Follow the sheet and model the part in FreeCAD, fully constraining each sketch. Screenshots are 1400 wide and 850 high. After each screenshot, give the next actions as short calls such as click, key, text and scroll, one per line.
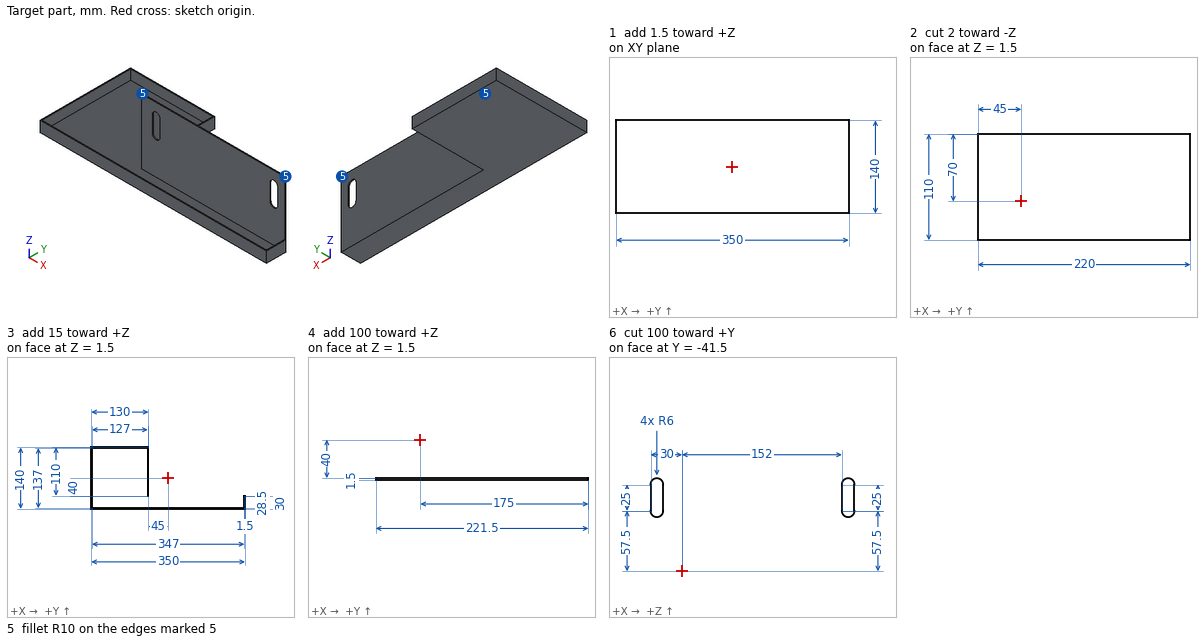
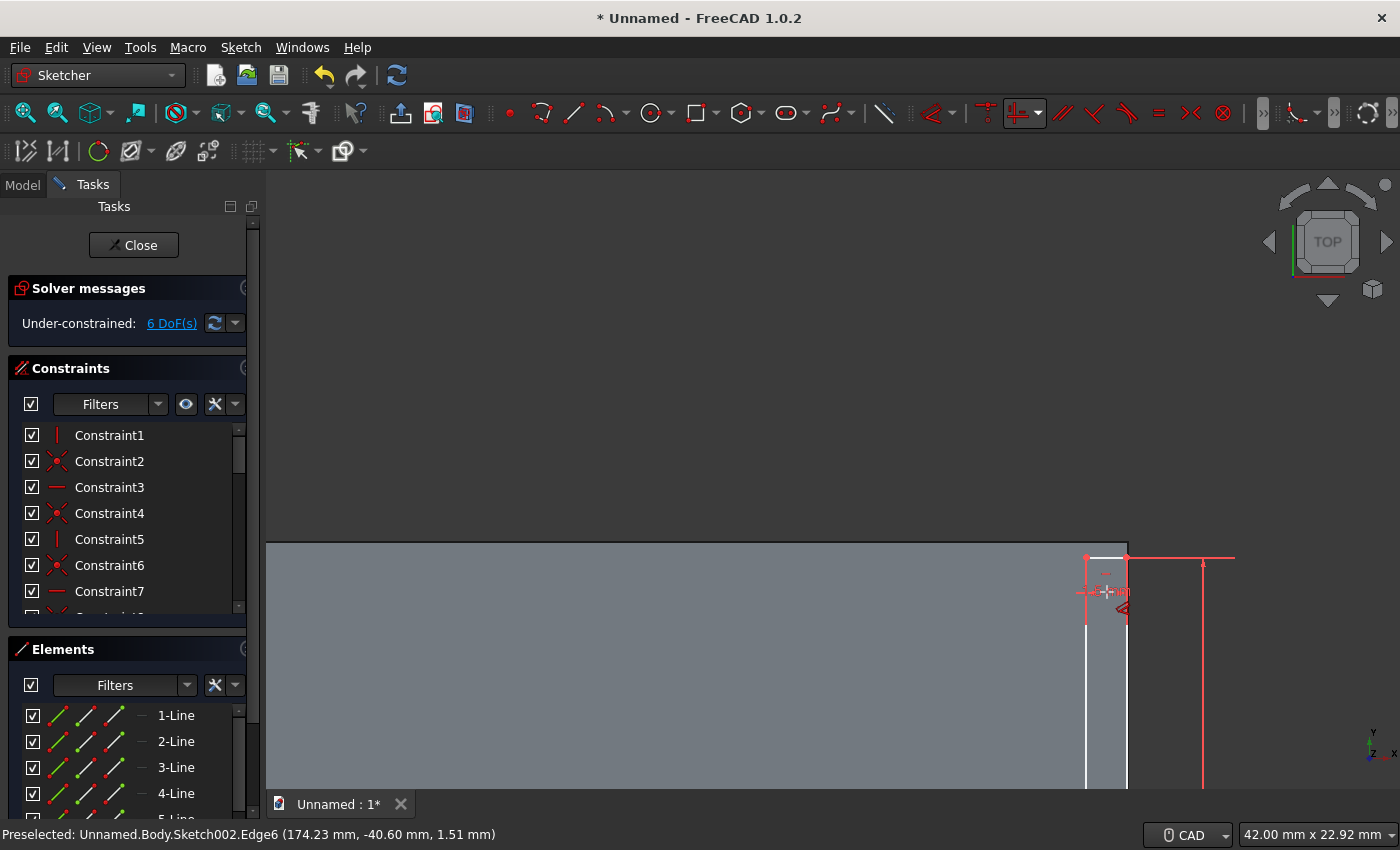
scroll(1114, 561, down, 13)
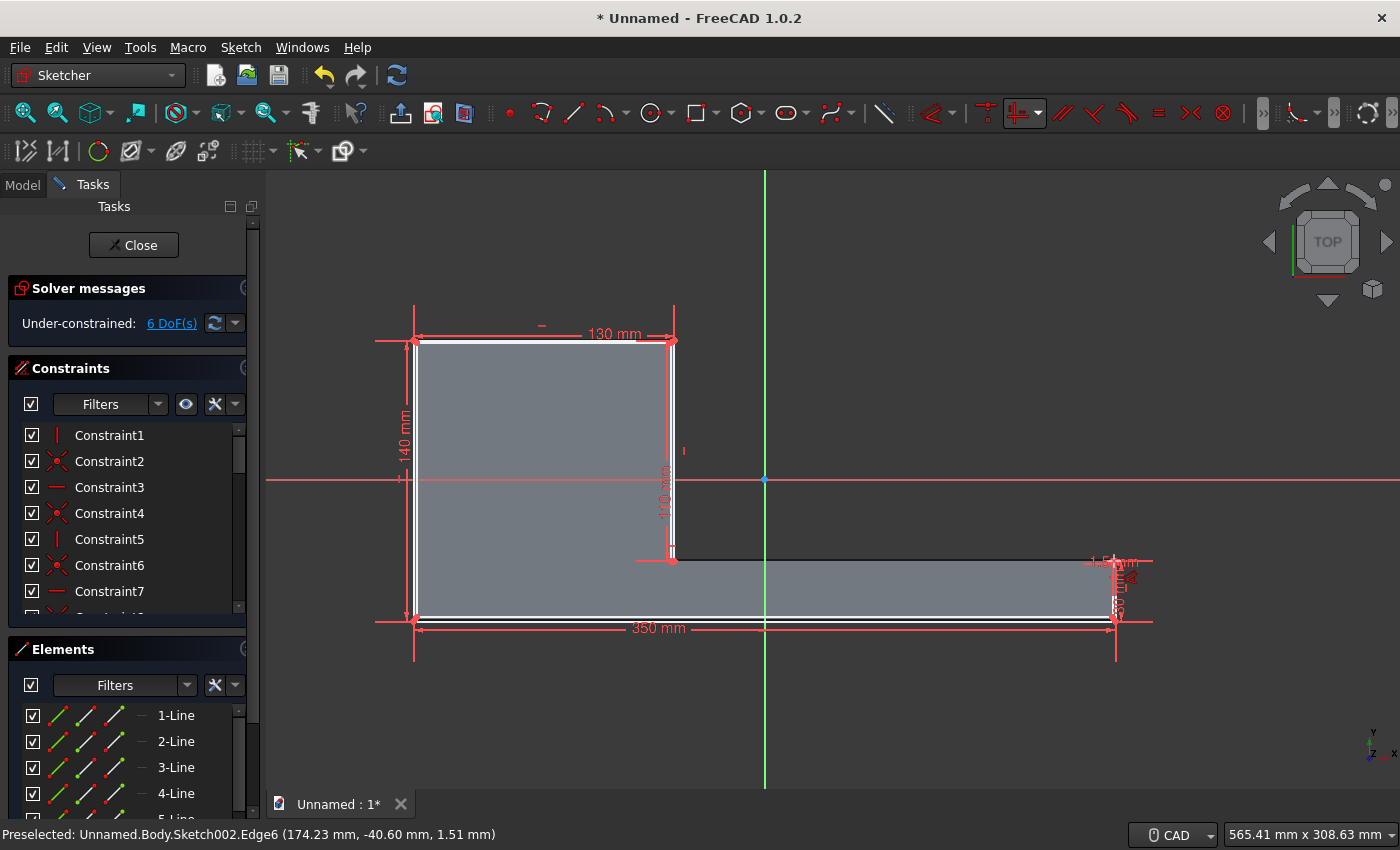
scroll(904, 617, up, 7)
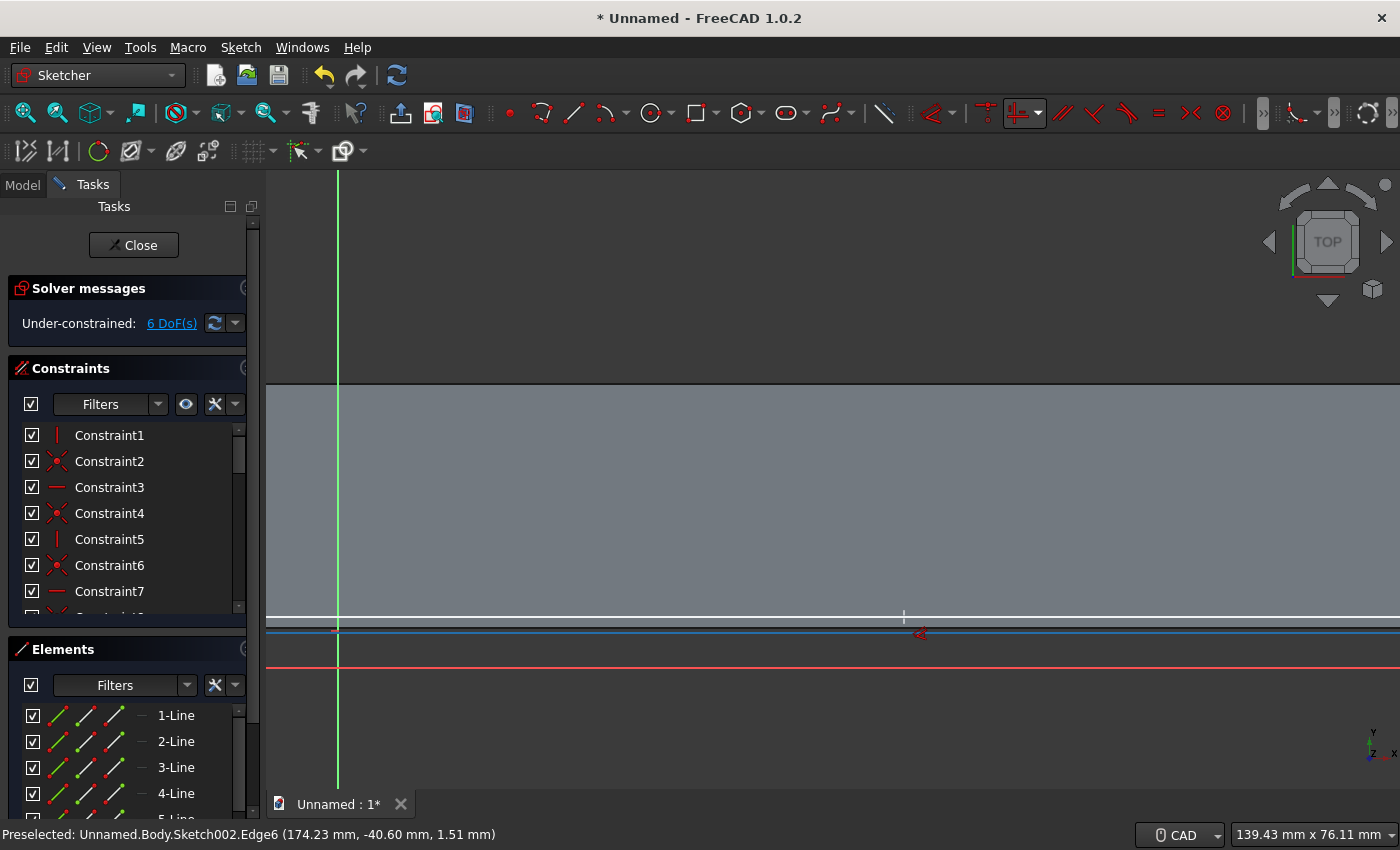
click(902, 617)
click(764, 651)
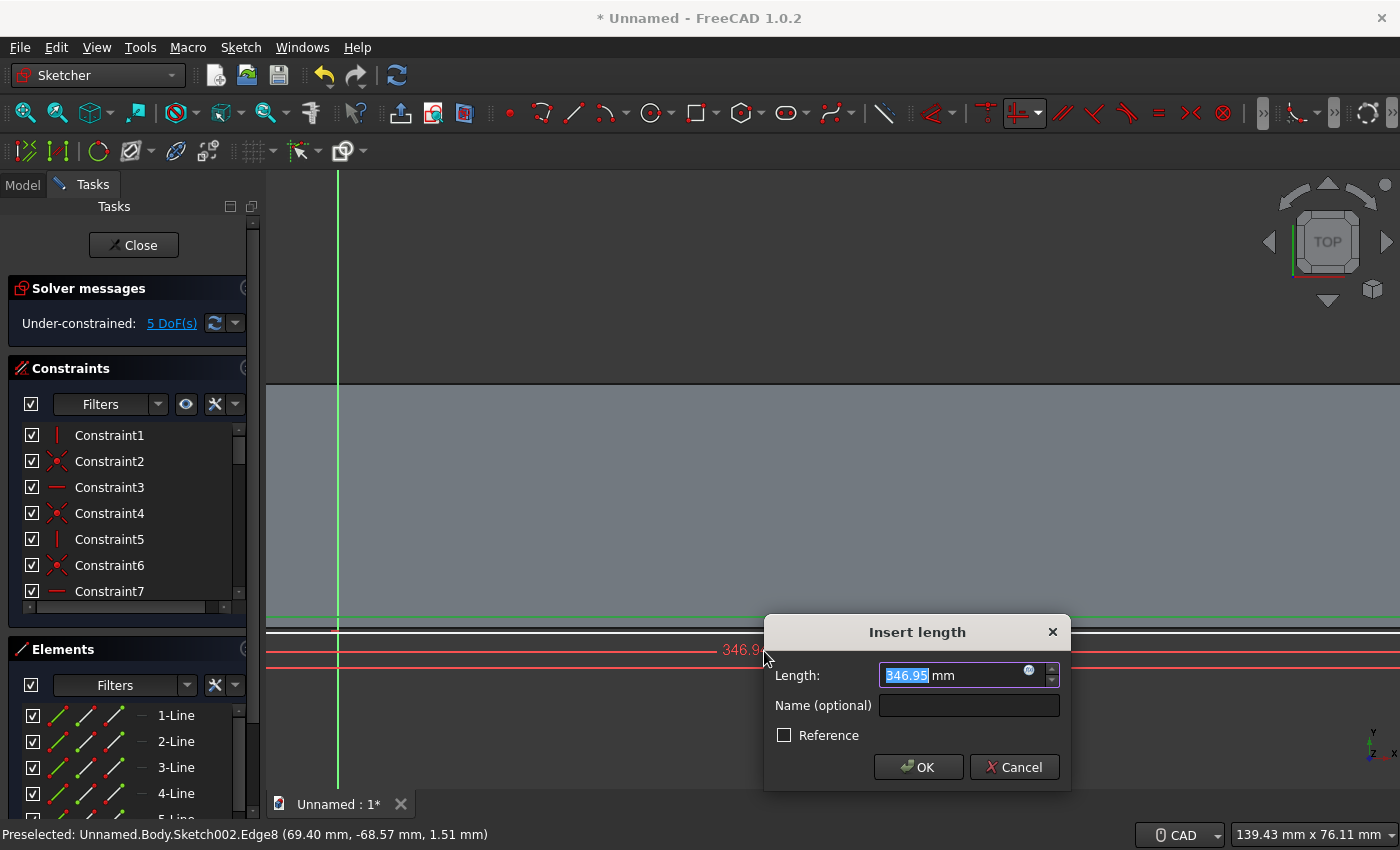
text(347)
key(Return)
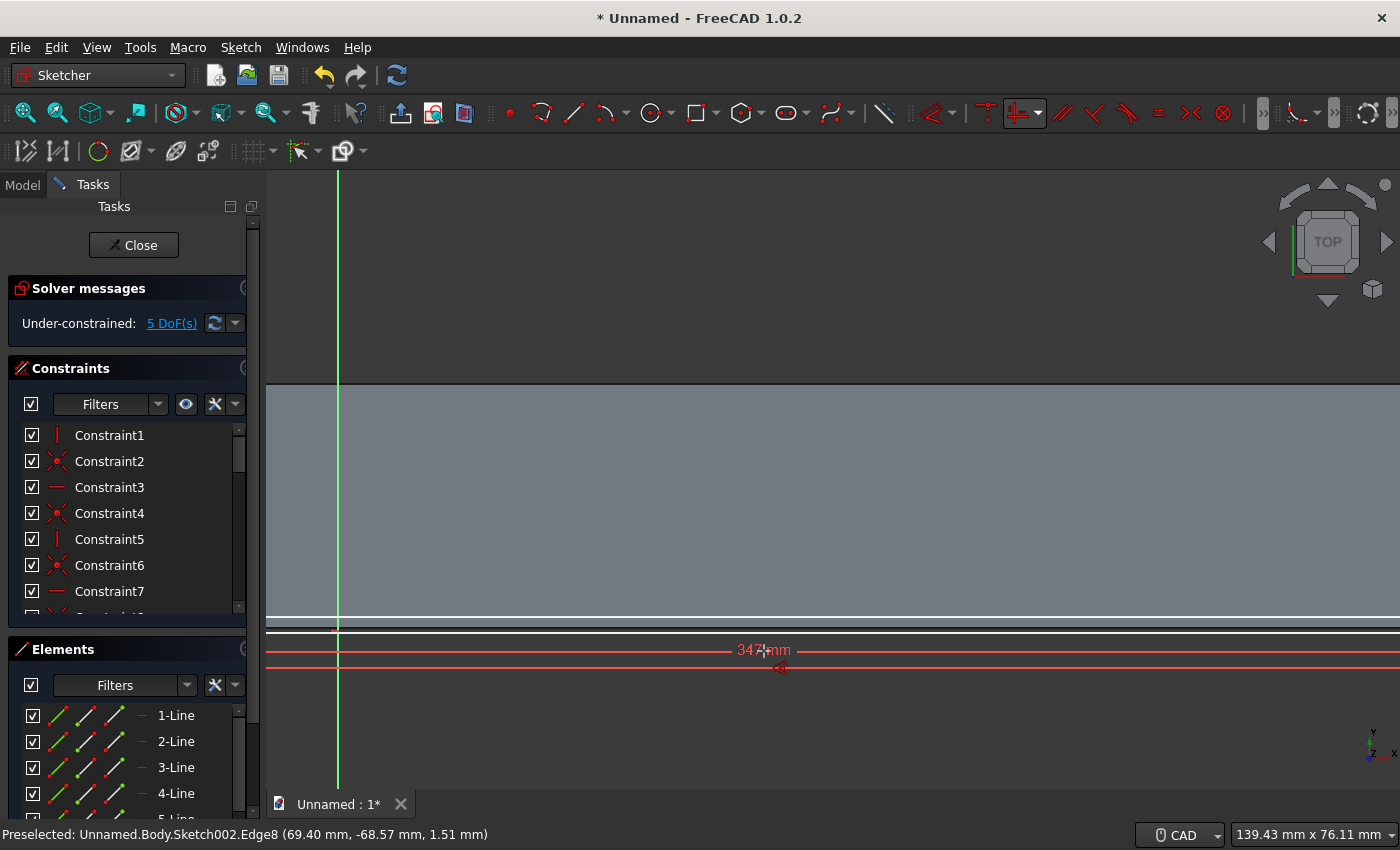
scroll(904, 617, down, 7)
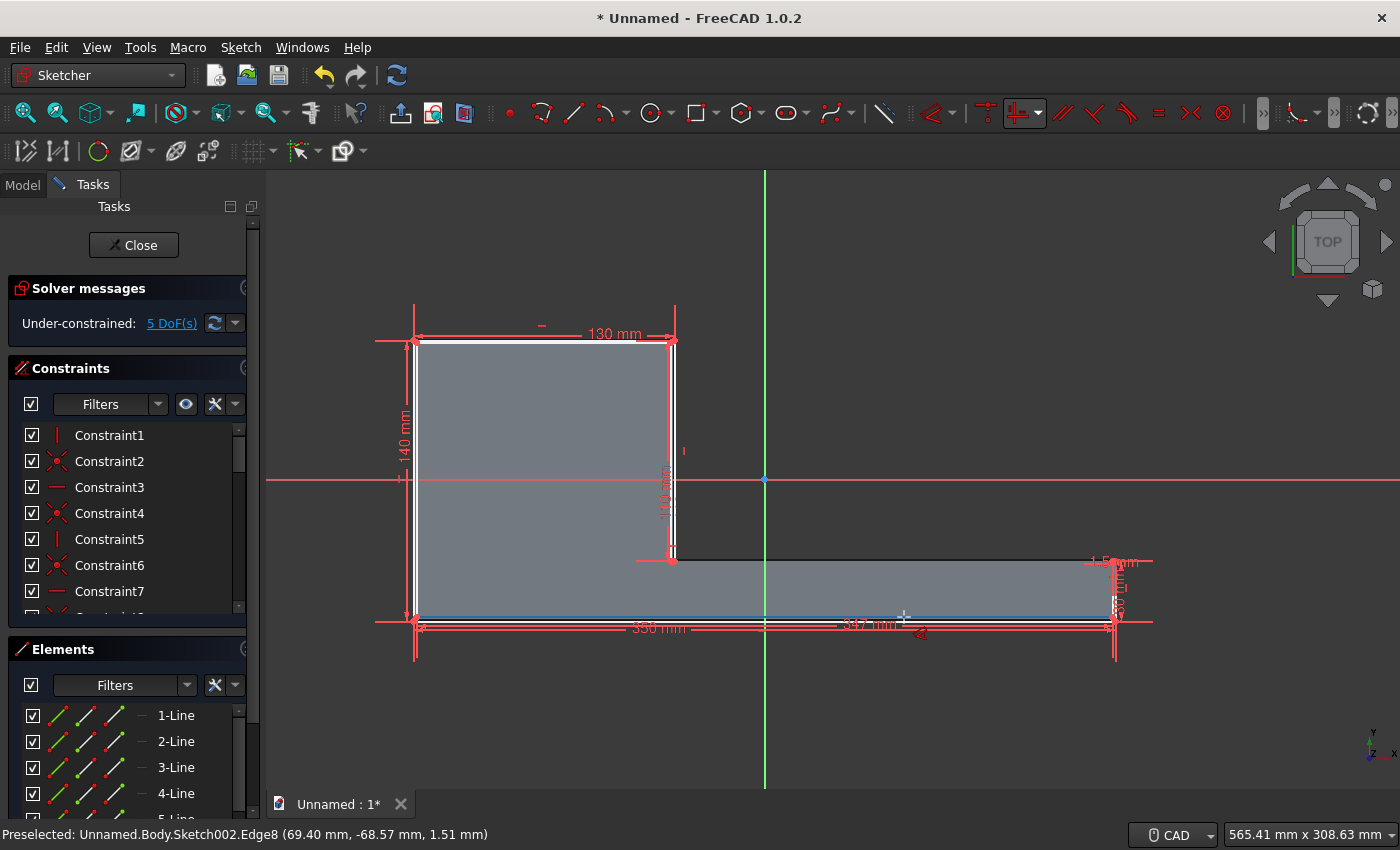
scroll(417, 535, up, 8)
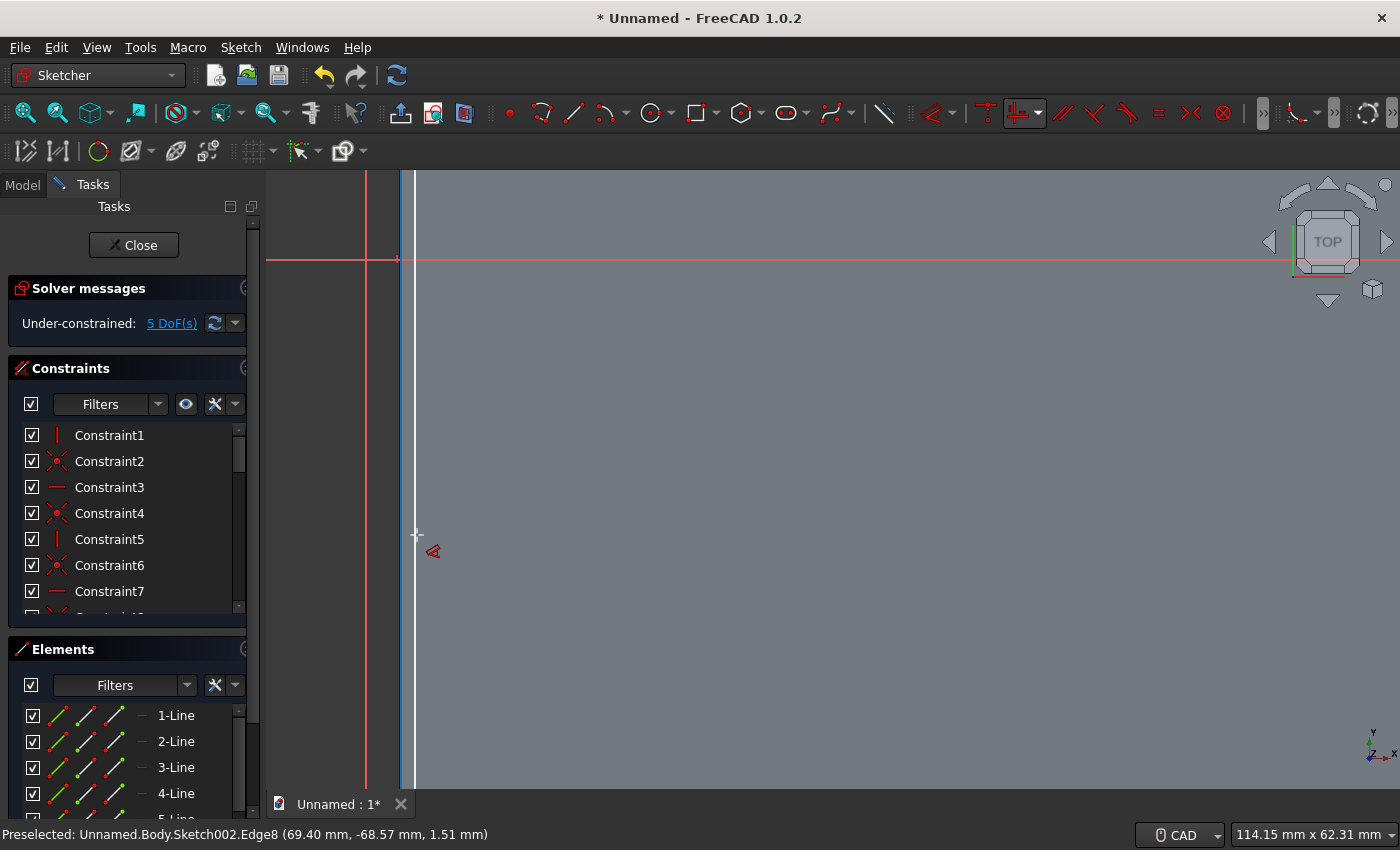
click(415, 533)
click(381, 480)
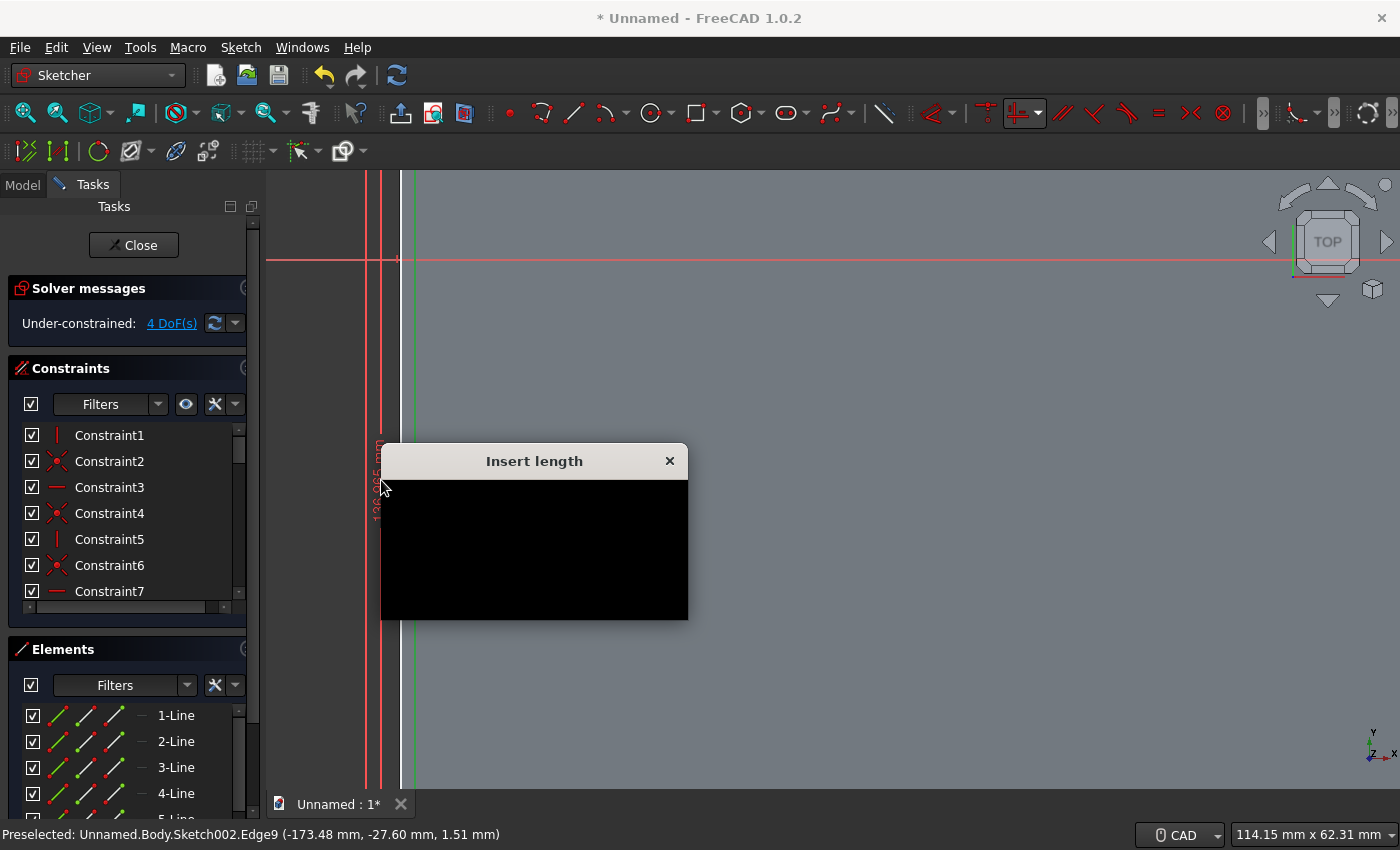
text(137)
key(Return)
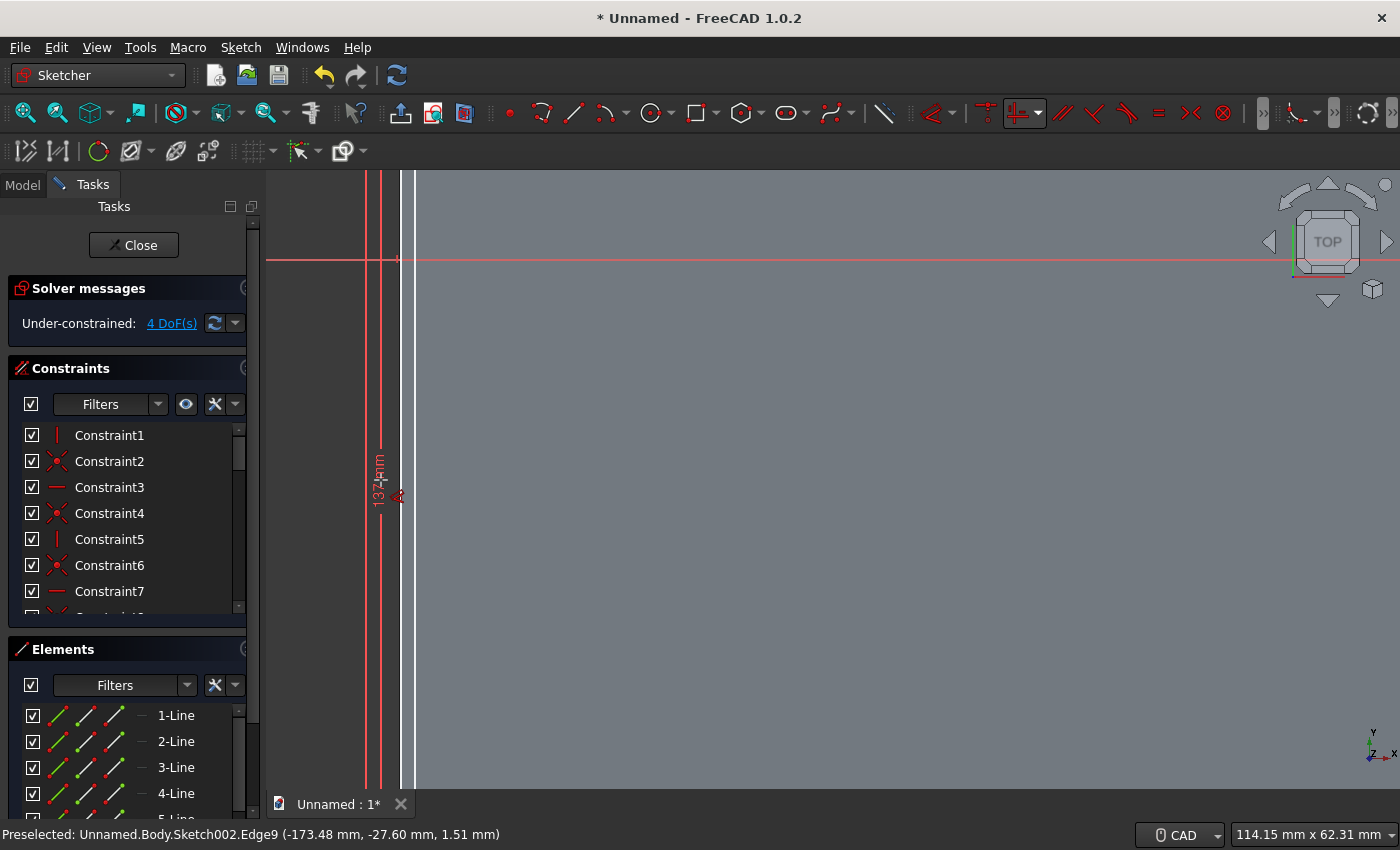
scroll(417, 535, down, 8)